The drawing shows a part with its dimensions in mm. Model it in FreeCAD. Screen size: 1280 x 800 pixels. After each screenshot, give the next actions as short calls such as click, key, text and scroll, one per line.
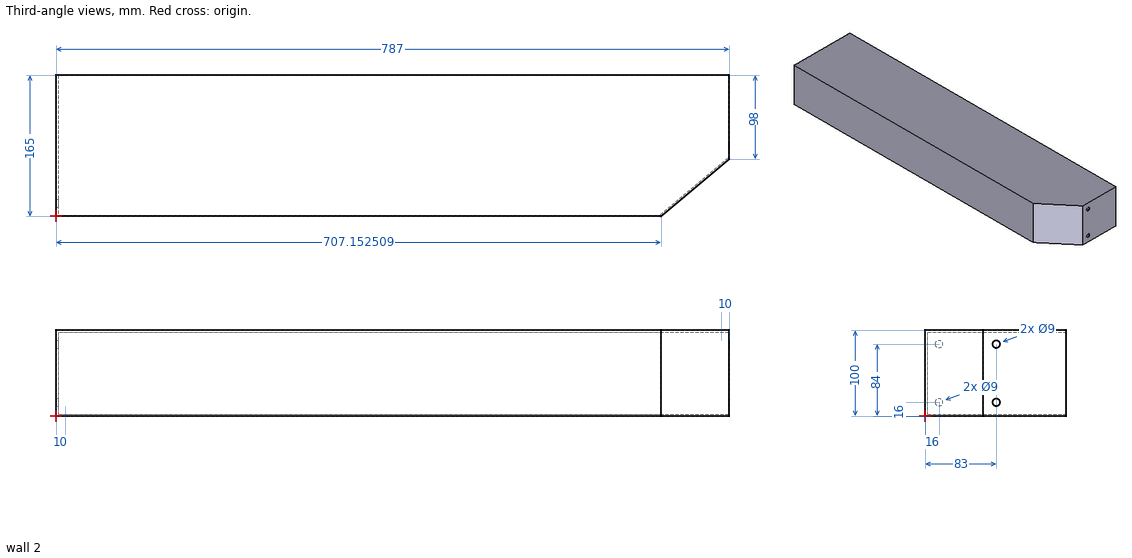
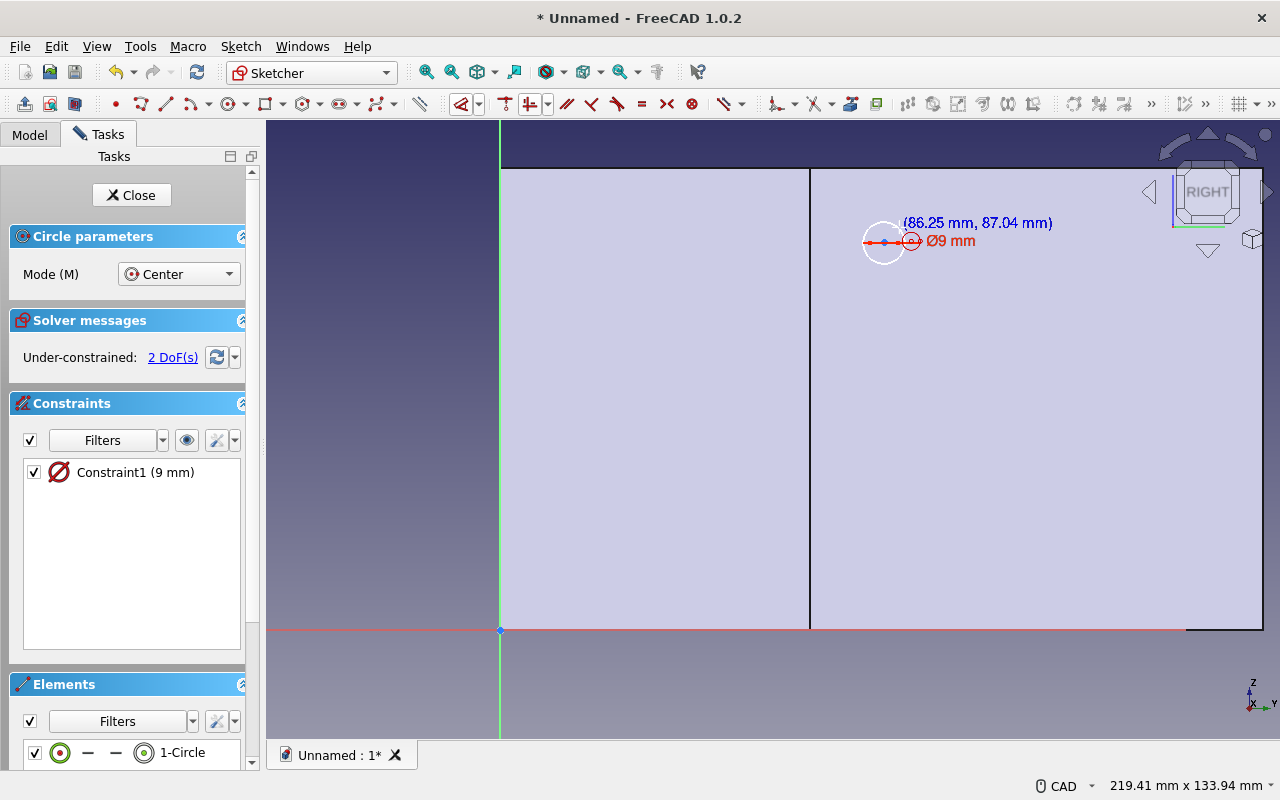
click(884, 556)
move(899, 542)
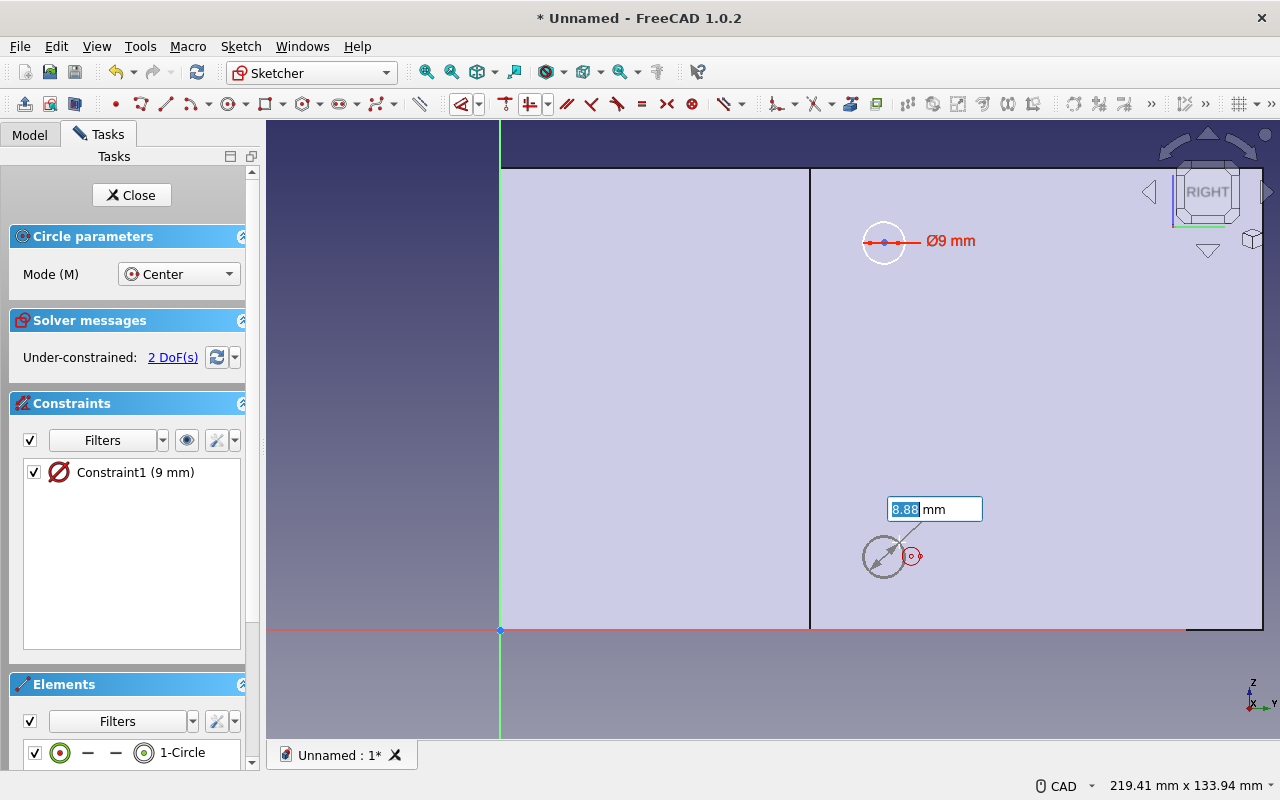
text(9)
key(Return)
key(Escape)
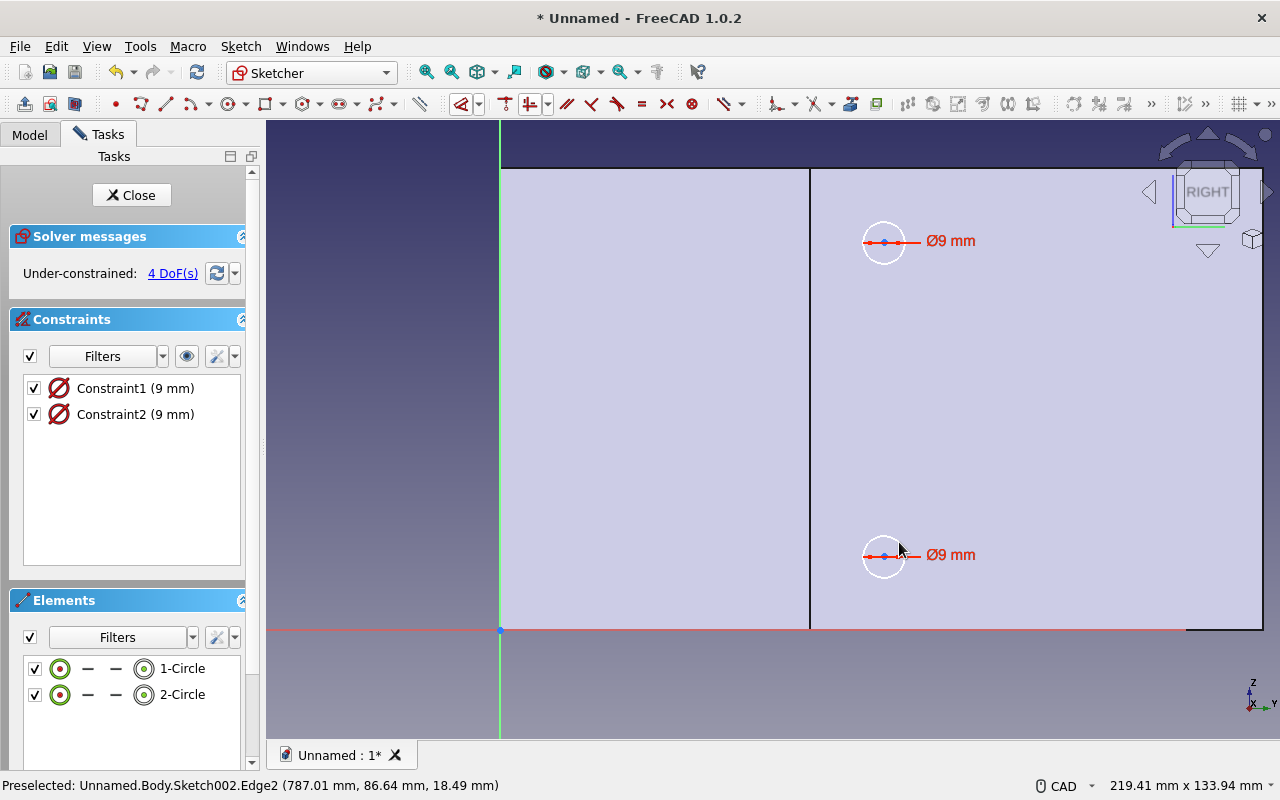
click(884, 243)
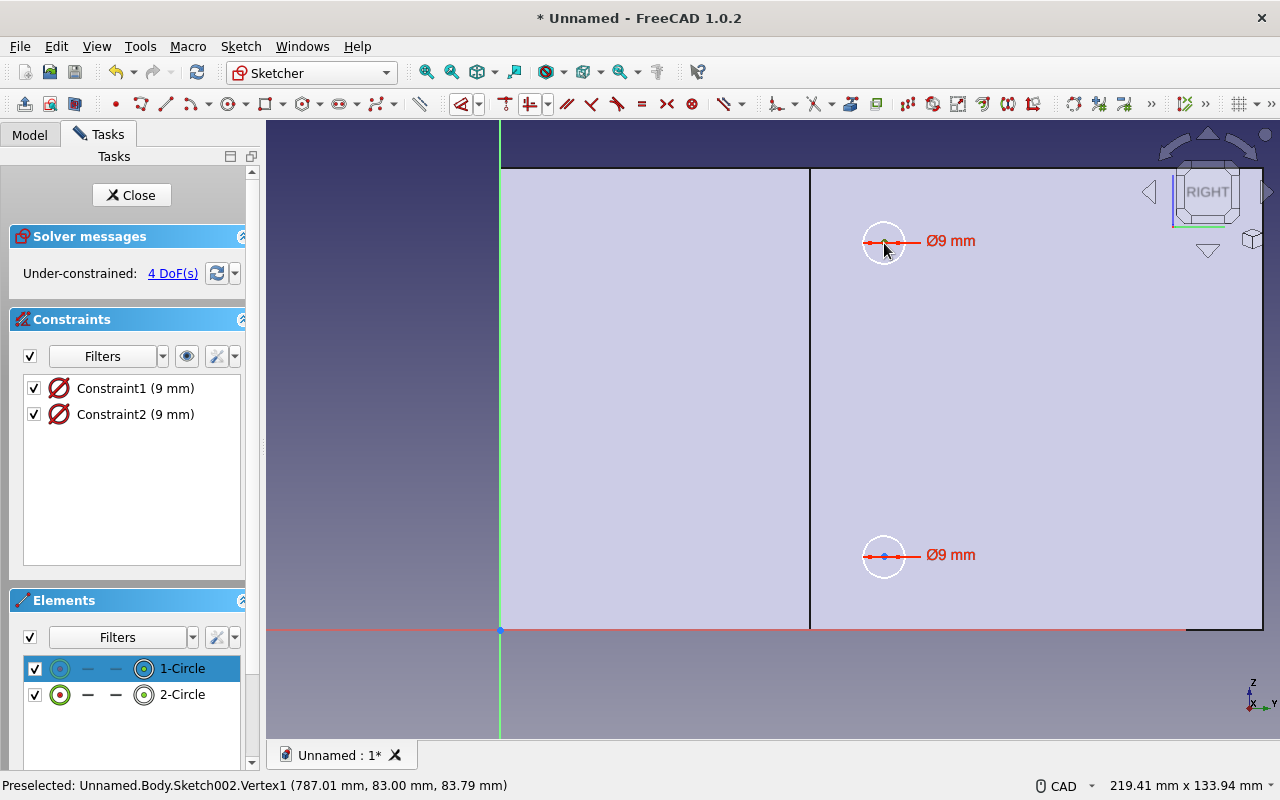
click(884, 557)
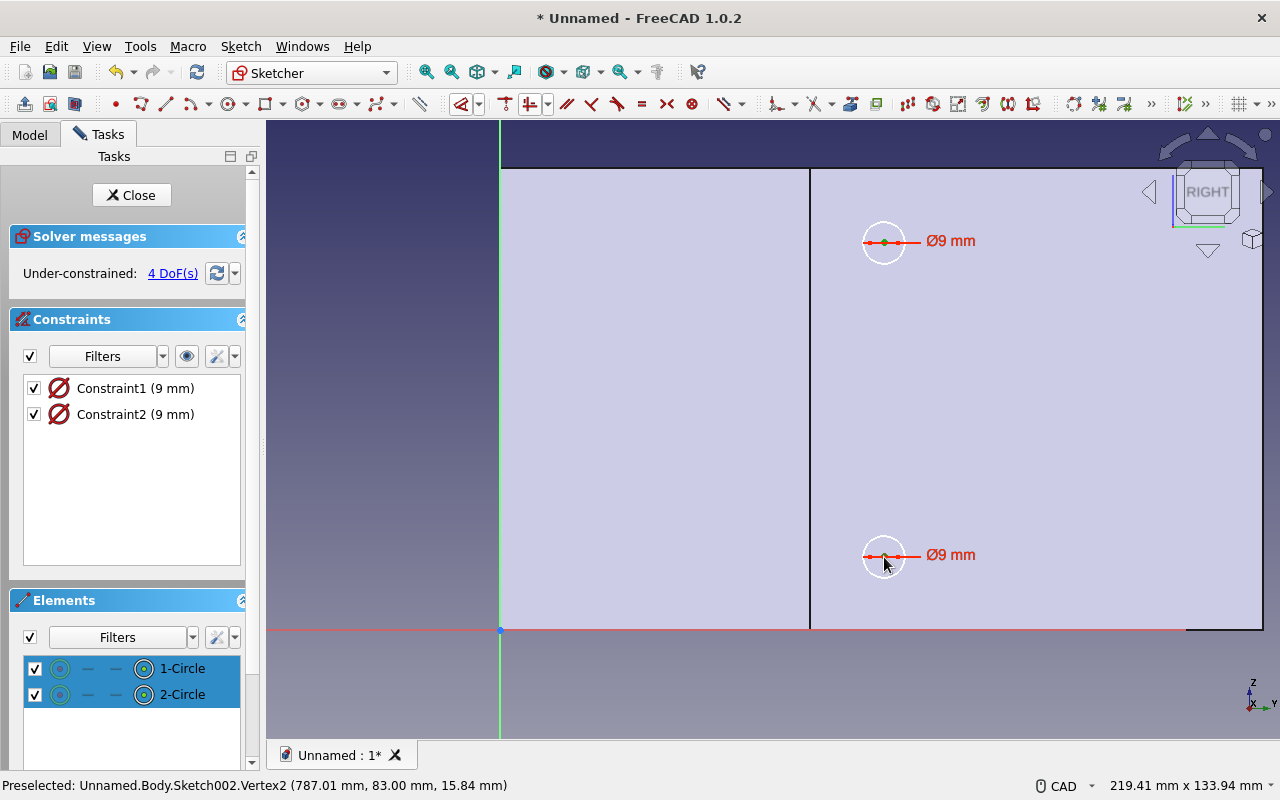
key(v)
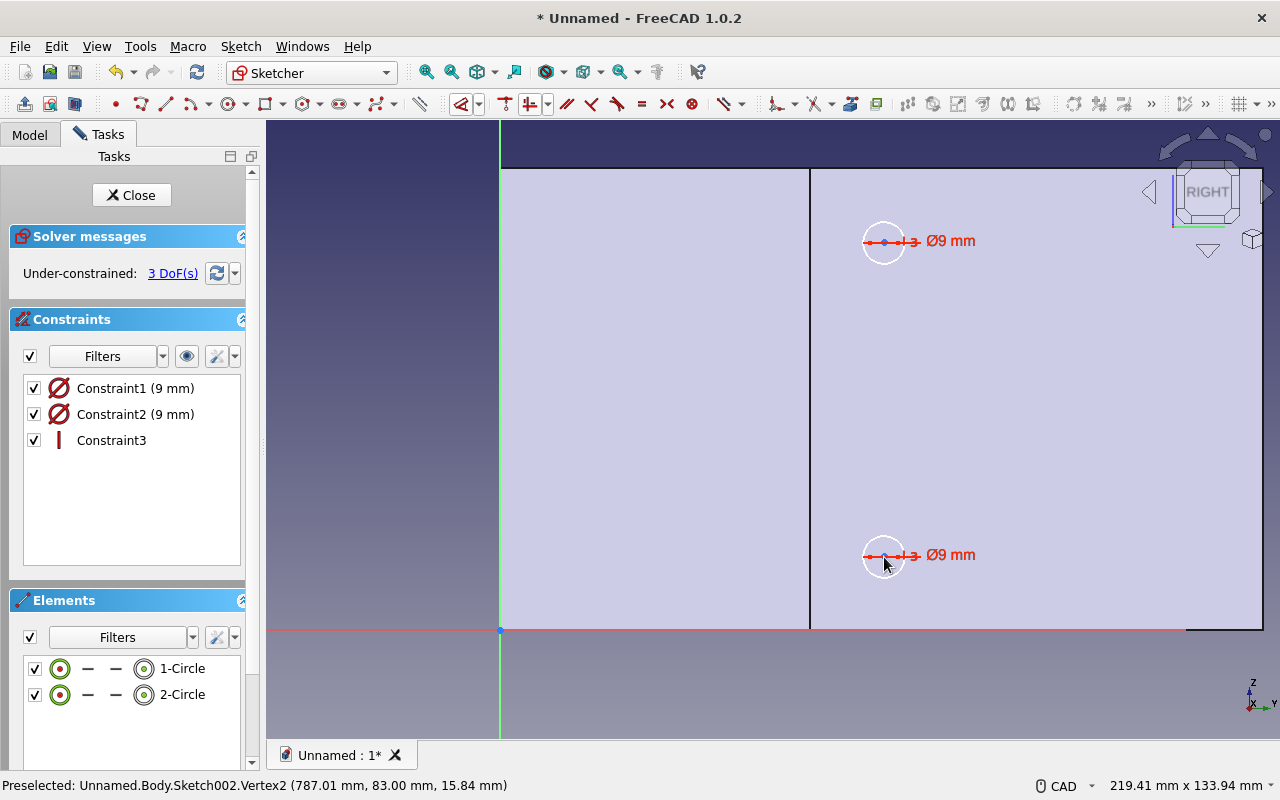
click(884, 243)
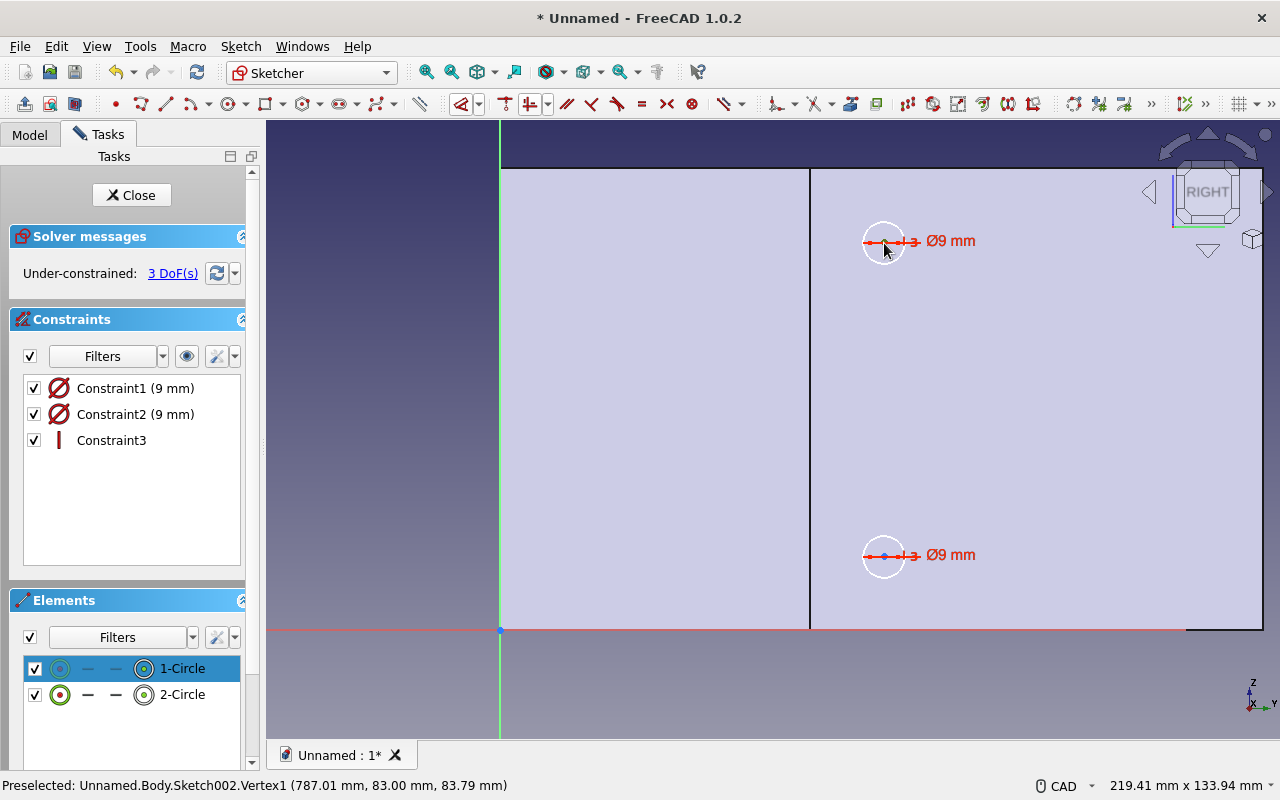
click(478, 104)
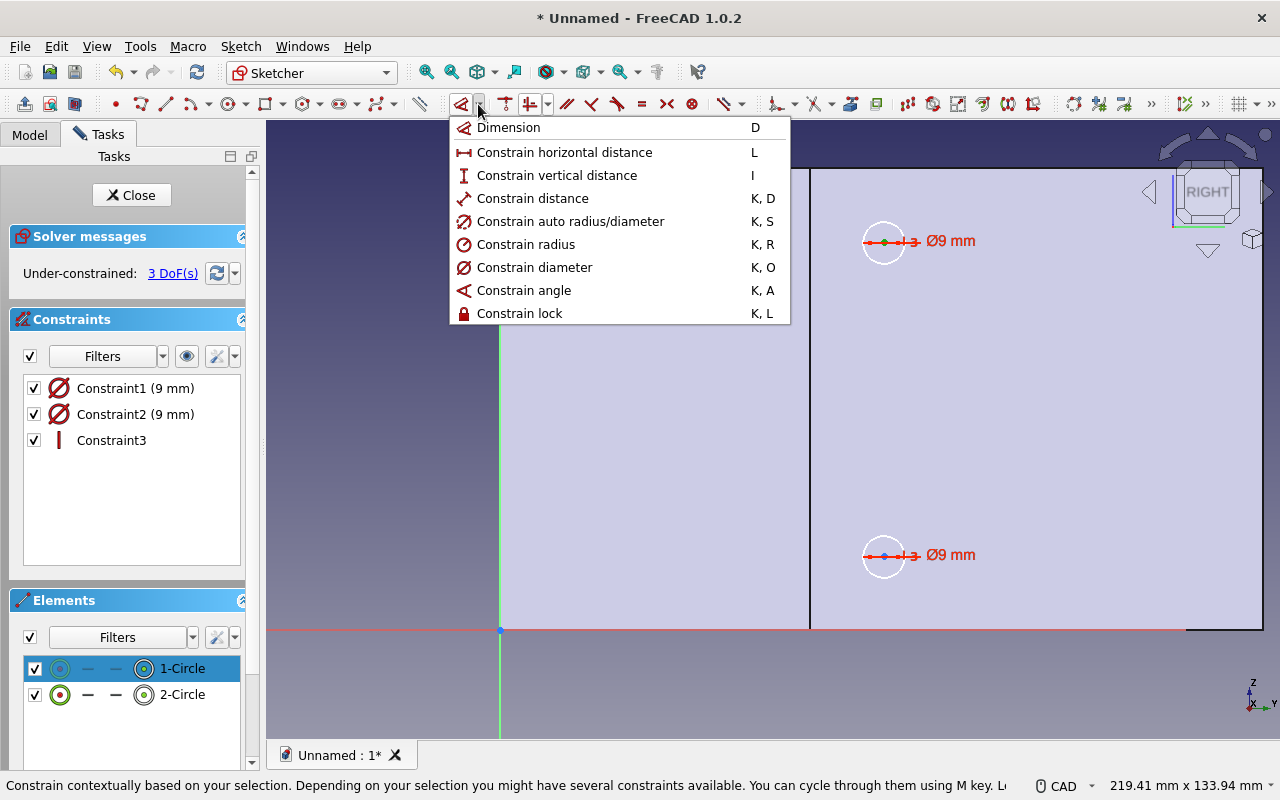
click(620, 152)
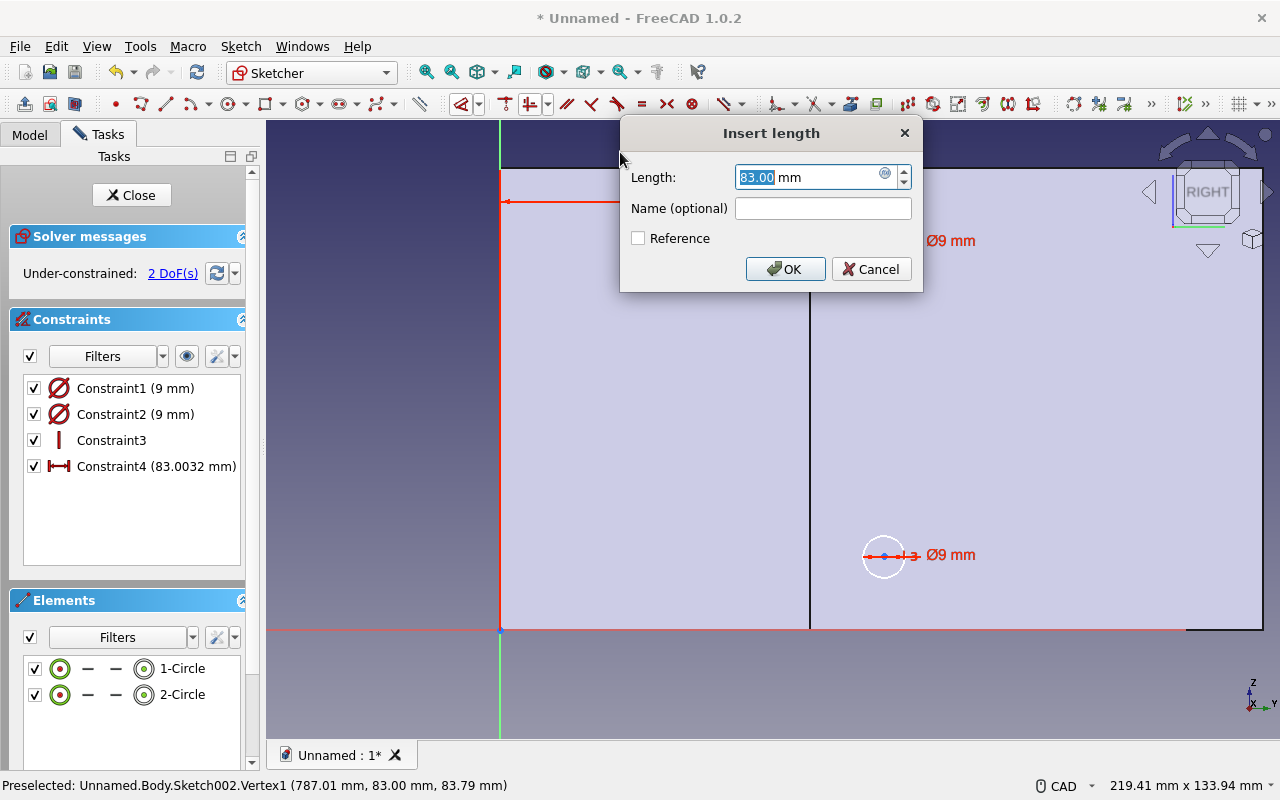
text(83)
key(Return)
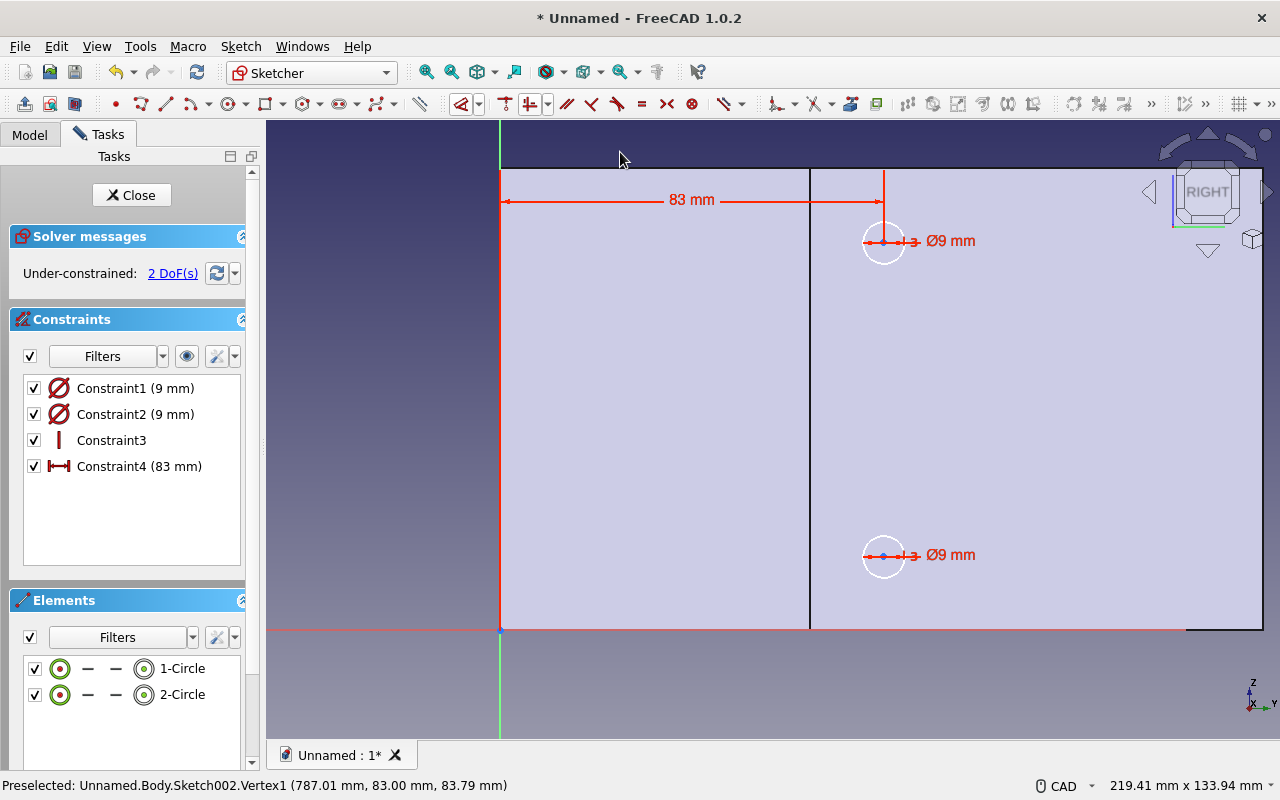
click(884, 243)